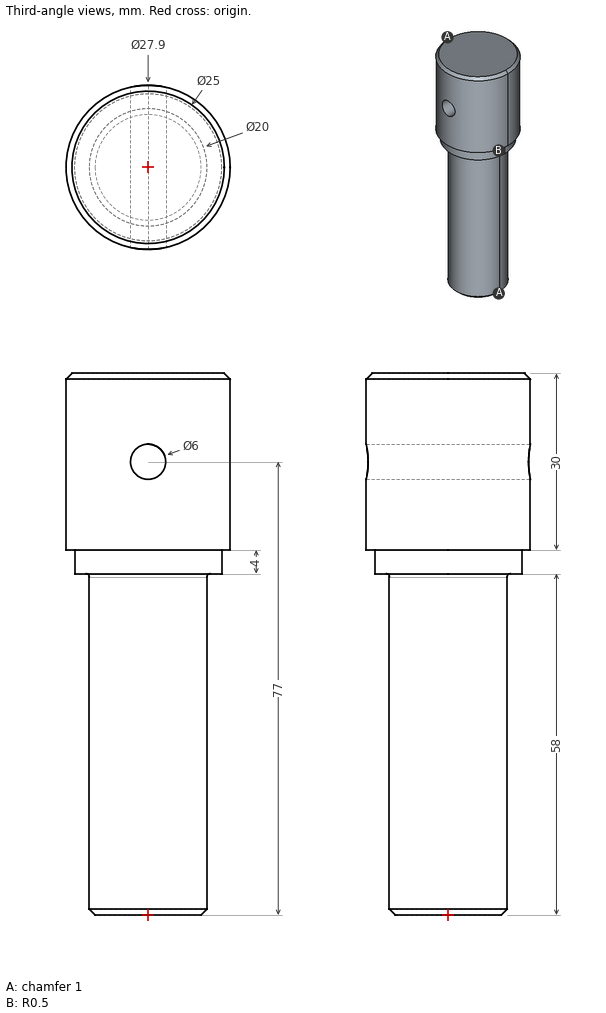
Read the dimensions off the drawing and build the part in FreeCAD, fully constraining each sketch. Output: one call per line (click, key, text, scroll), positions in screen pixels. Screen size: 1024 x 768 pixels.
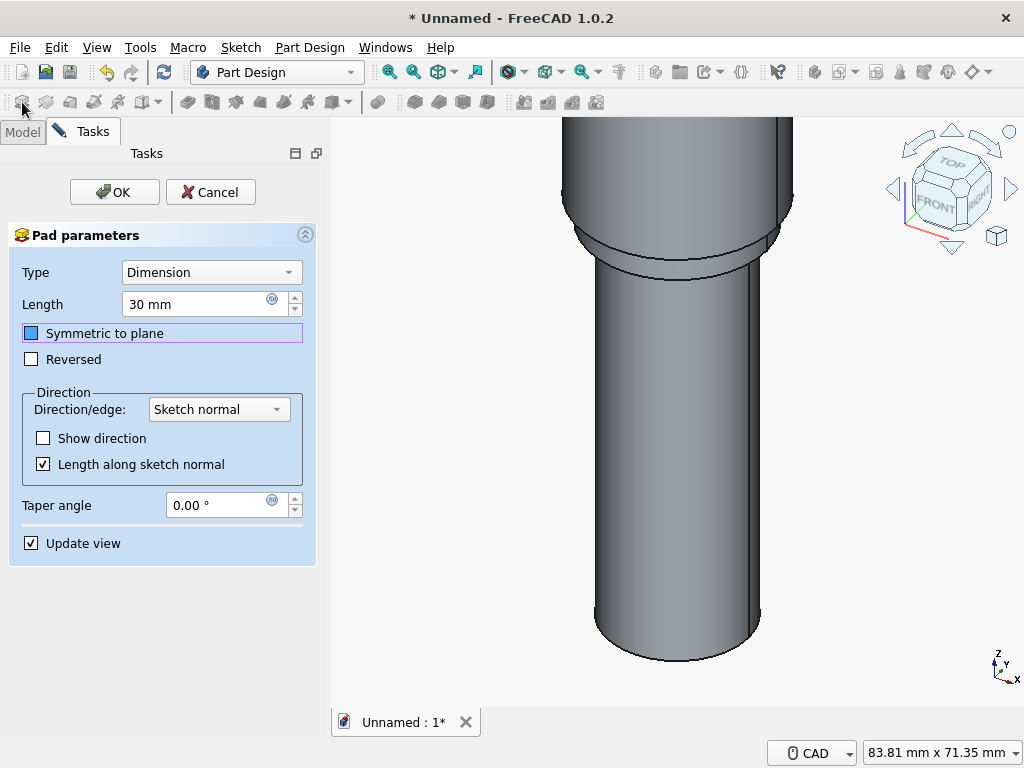
click(115, 192)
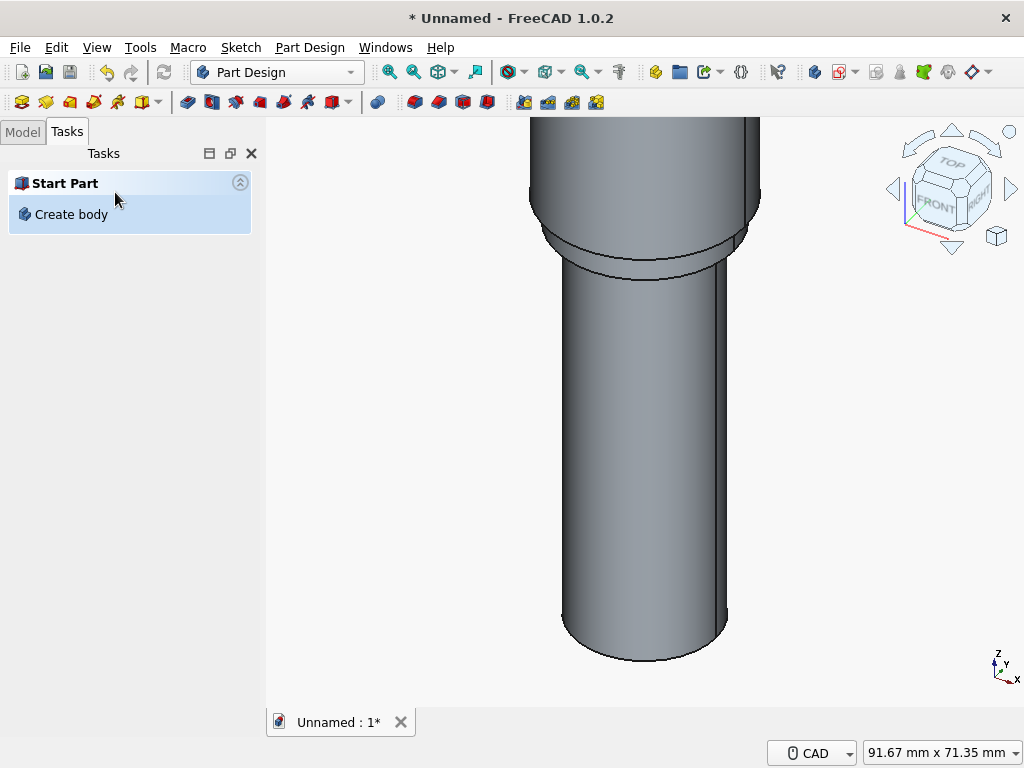
click(390, 72)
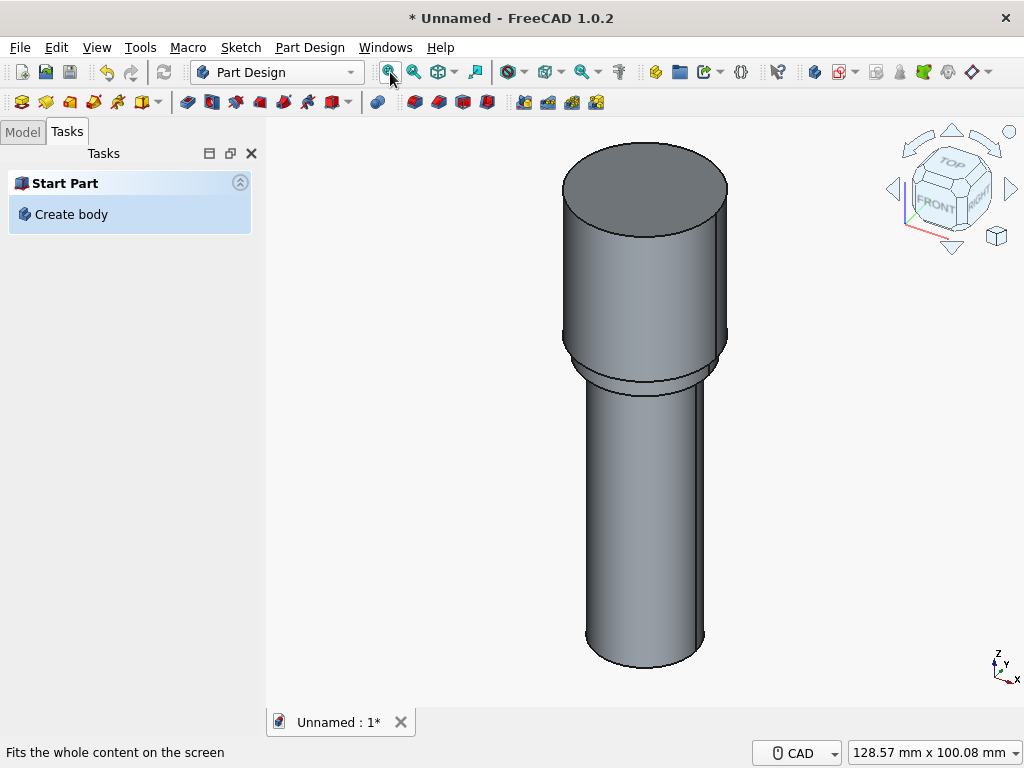
click(563, 194)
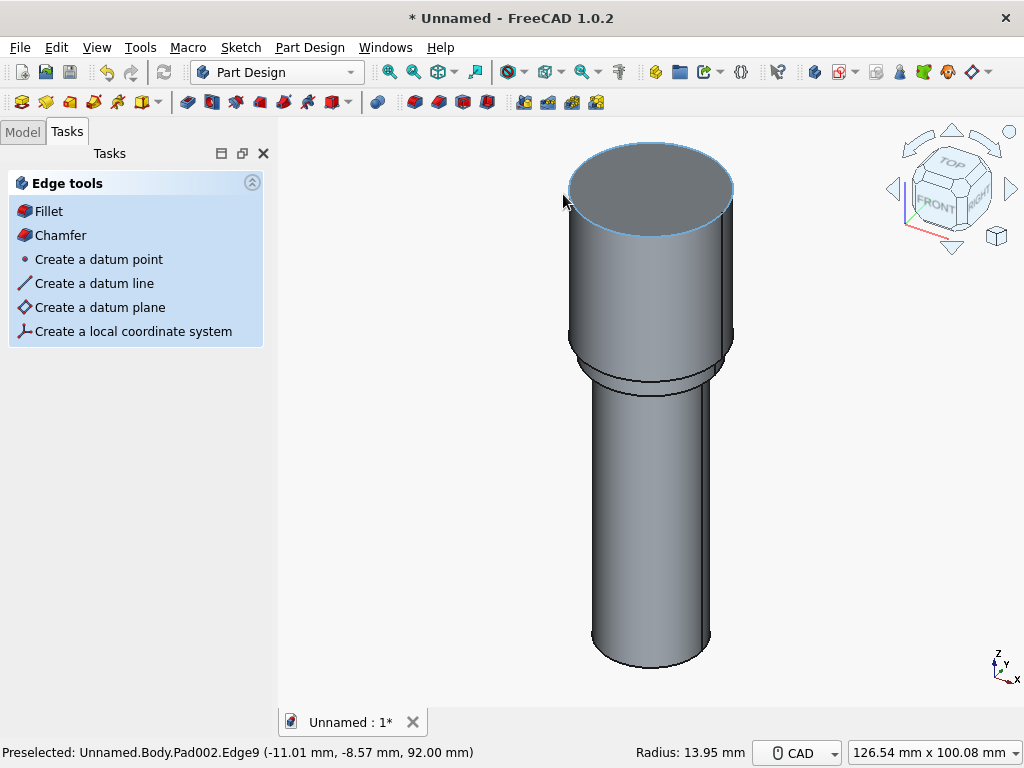
key(0)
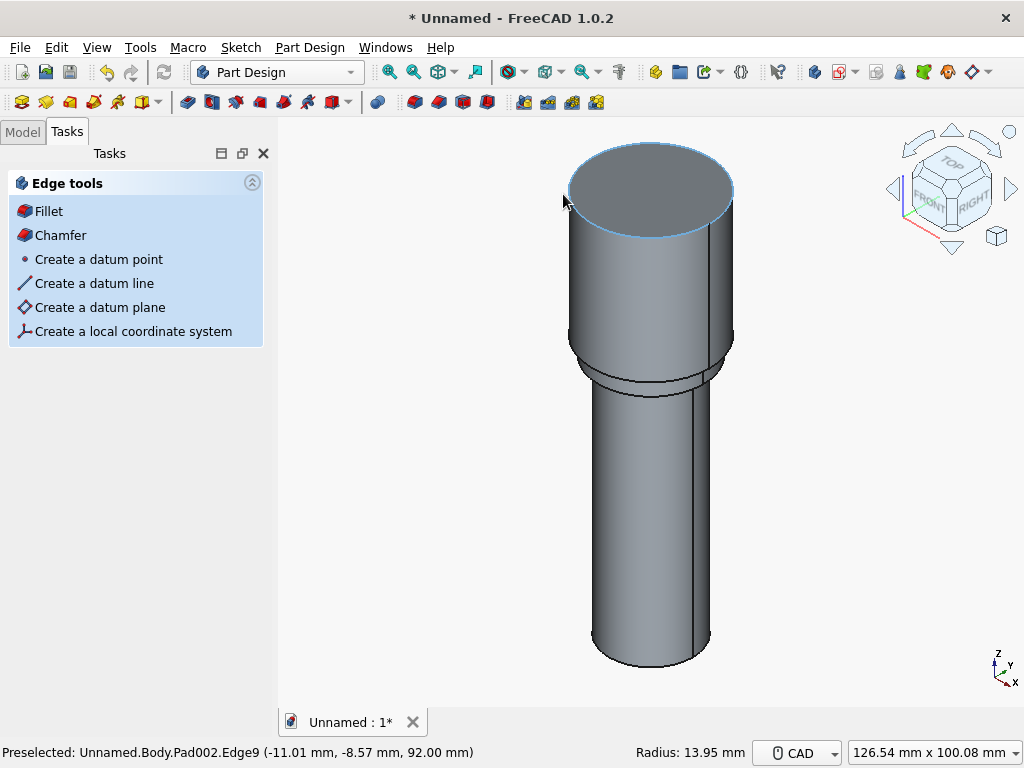
key(2)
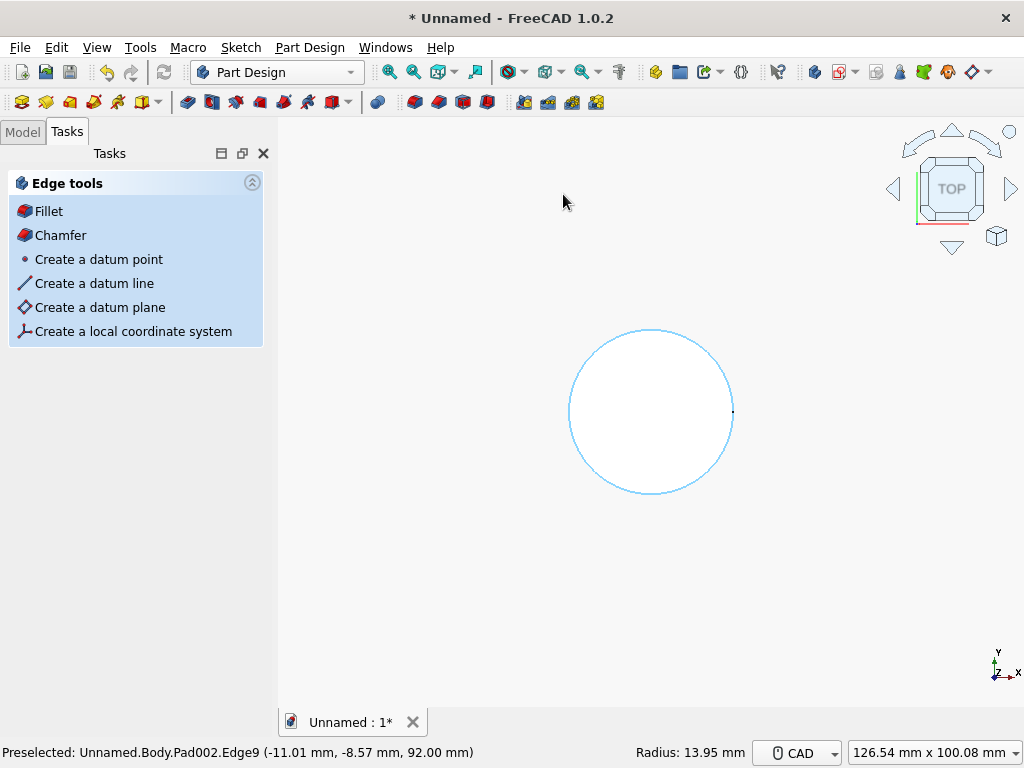
click(390, 72)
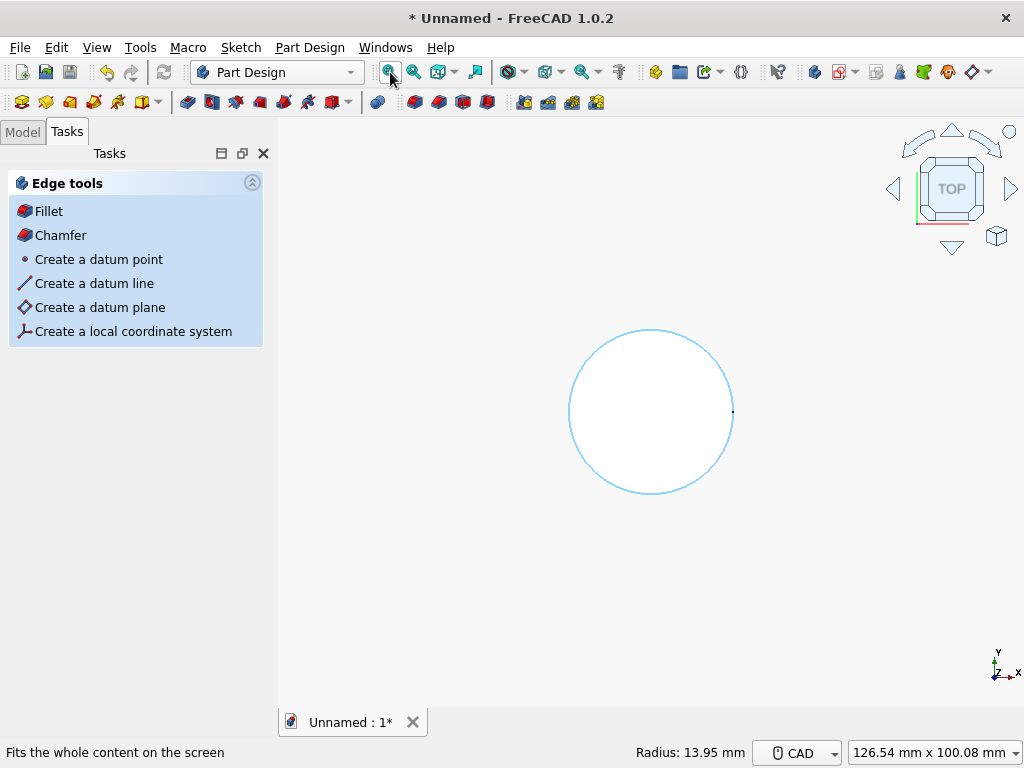
key(1)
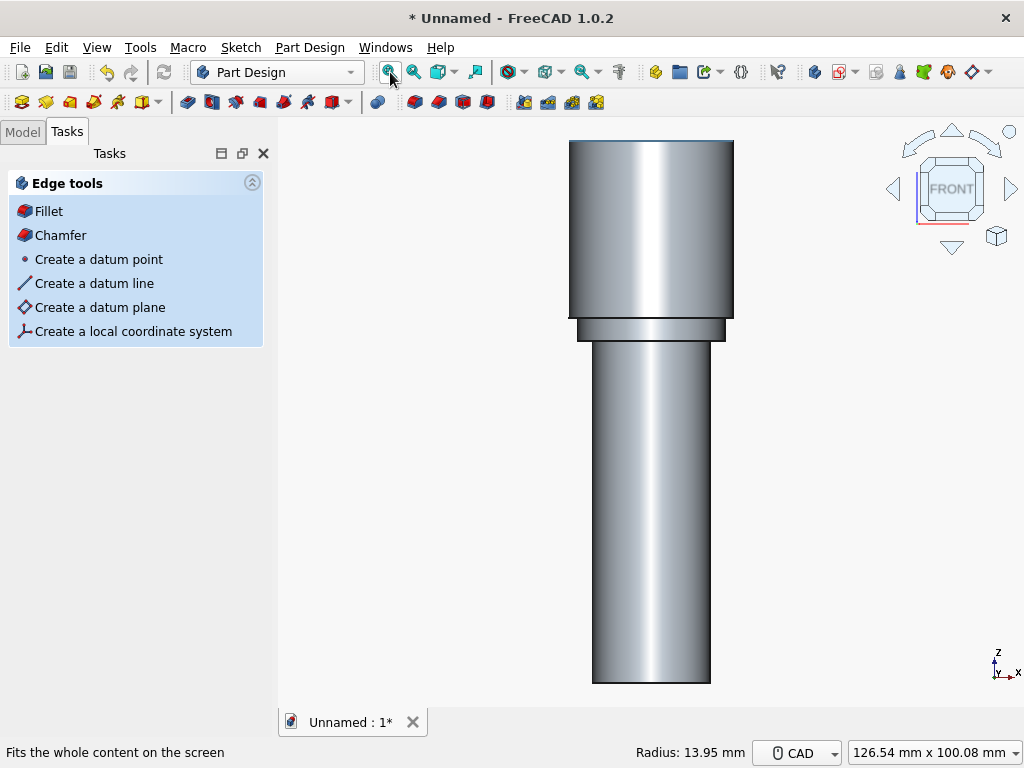
key(3)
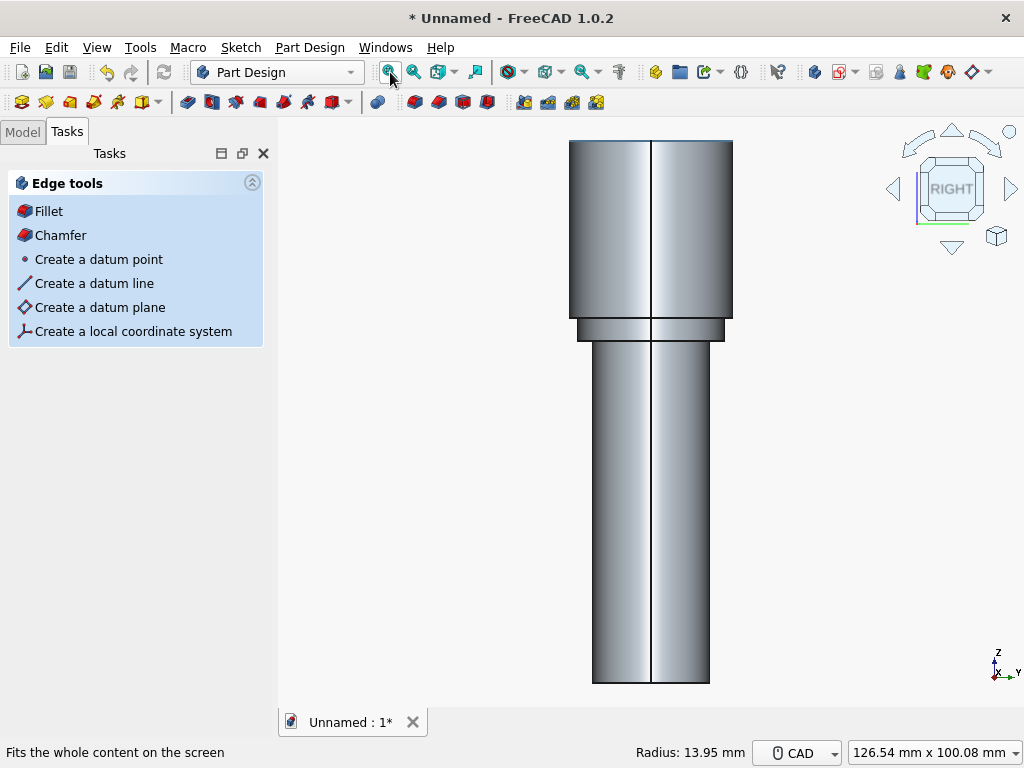
key(5)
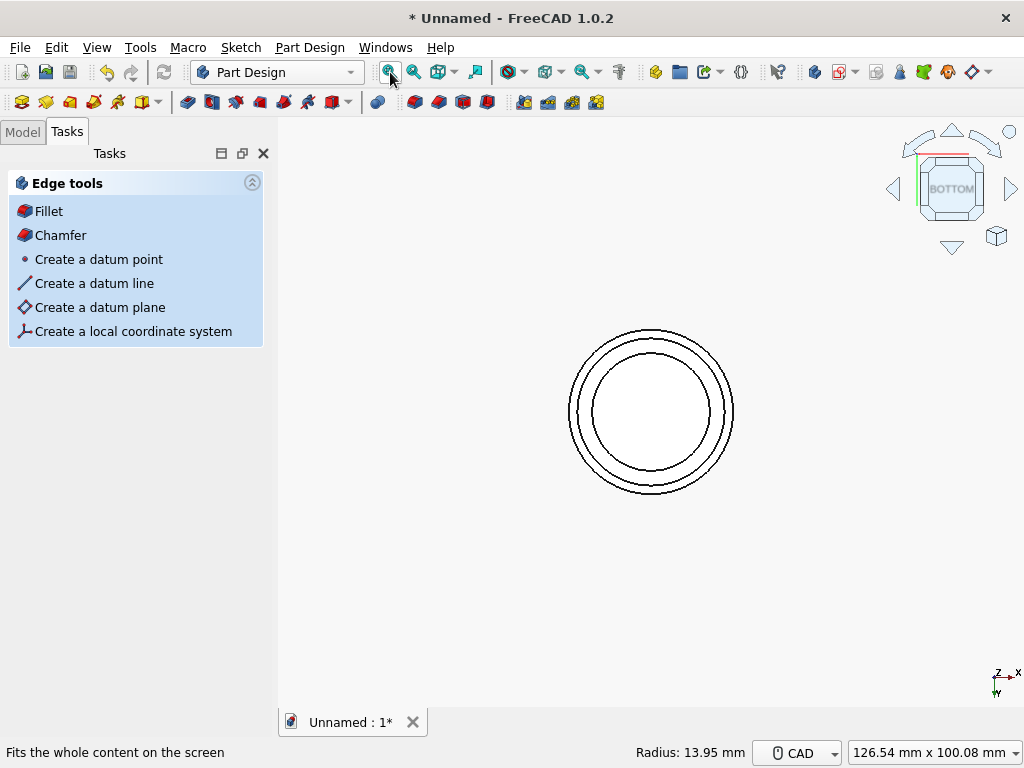
click(390, 72)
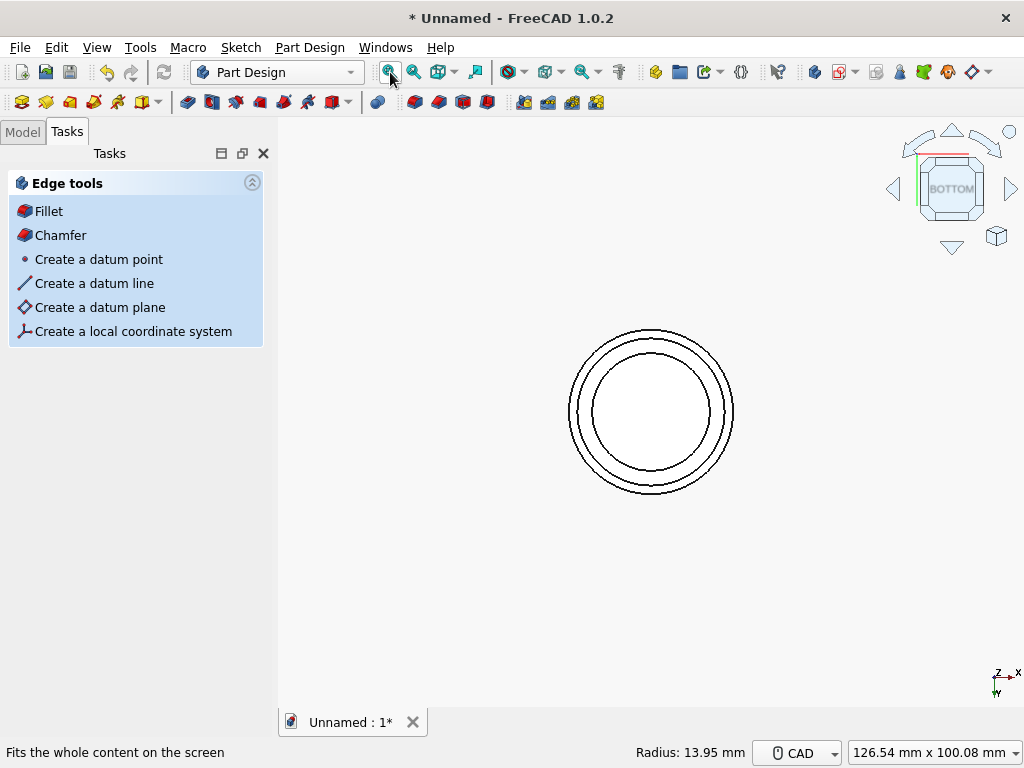
click(592, 411, ctrl)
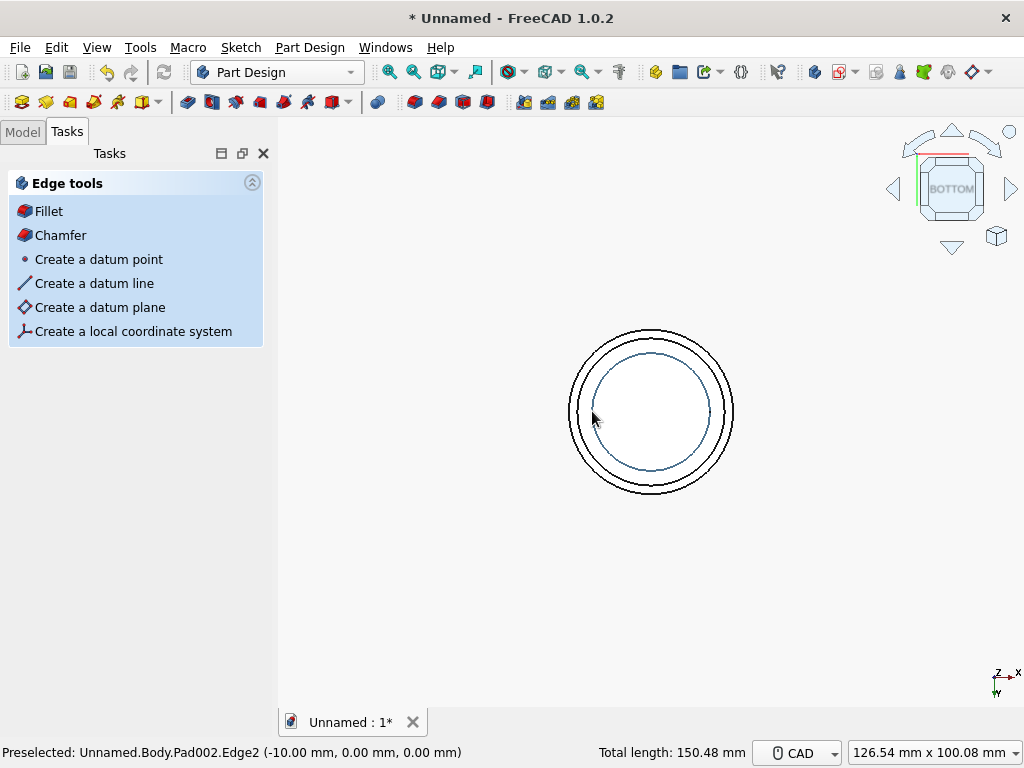
click(440, 102)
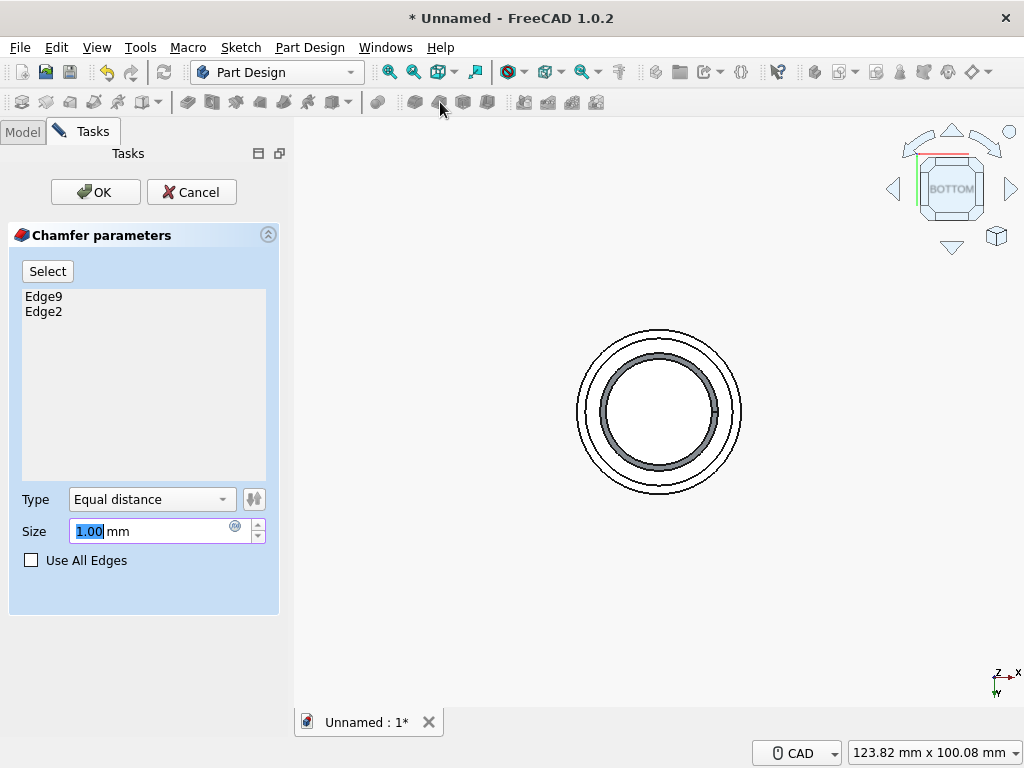
text(1)
key(Tab)